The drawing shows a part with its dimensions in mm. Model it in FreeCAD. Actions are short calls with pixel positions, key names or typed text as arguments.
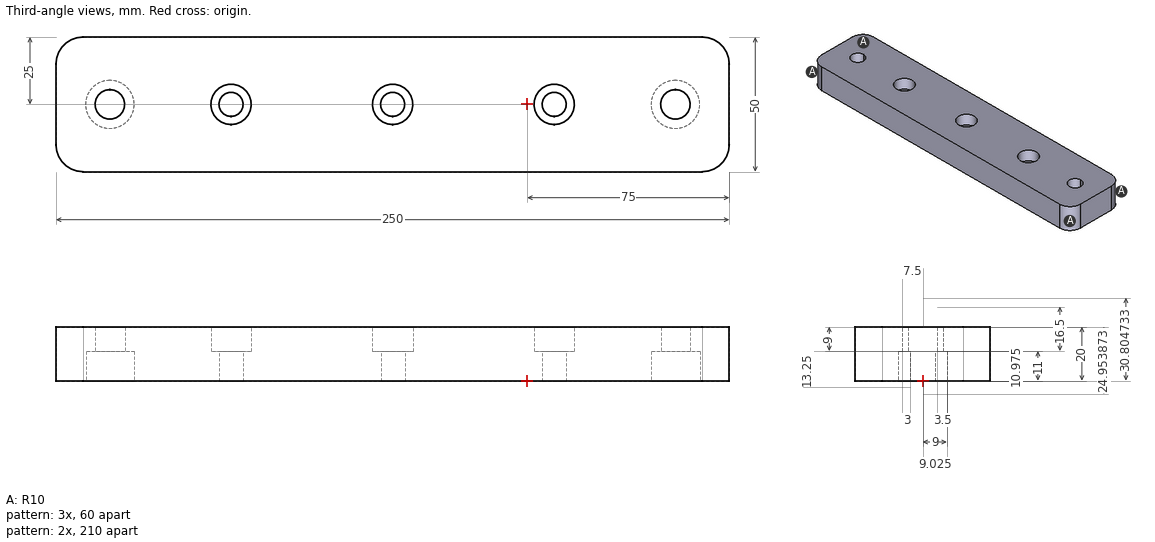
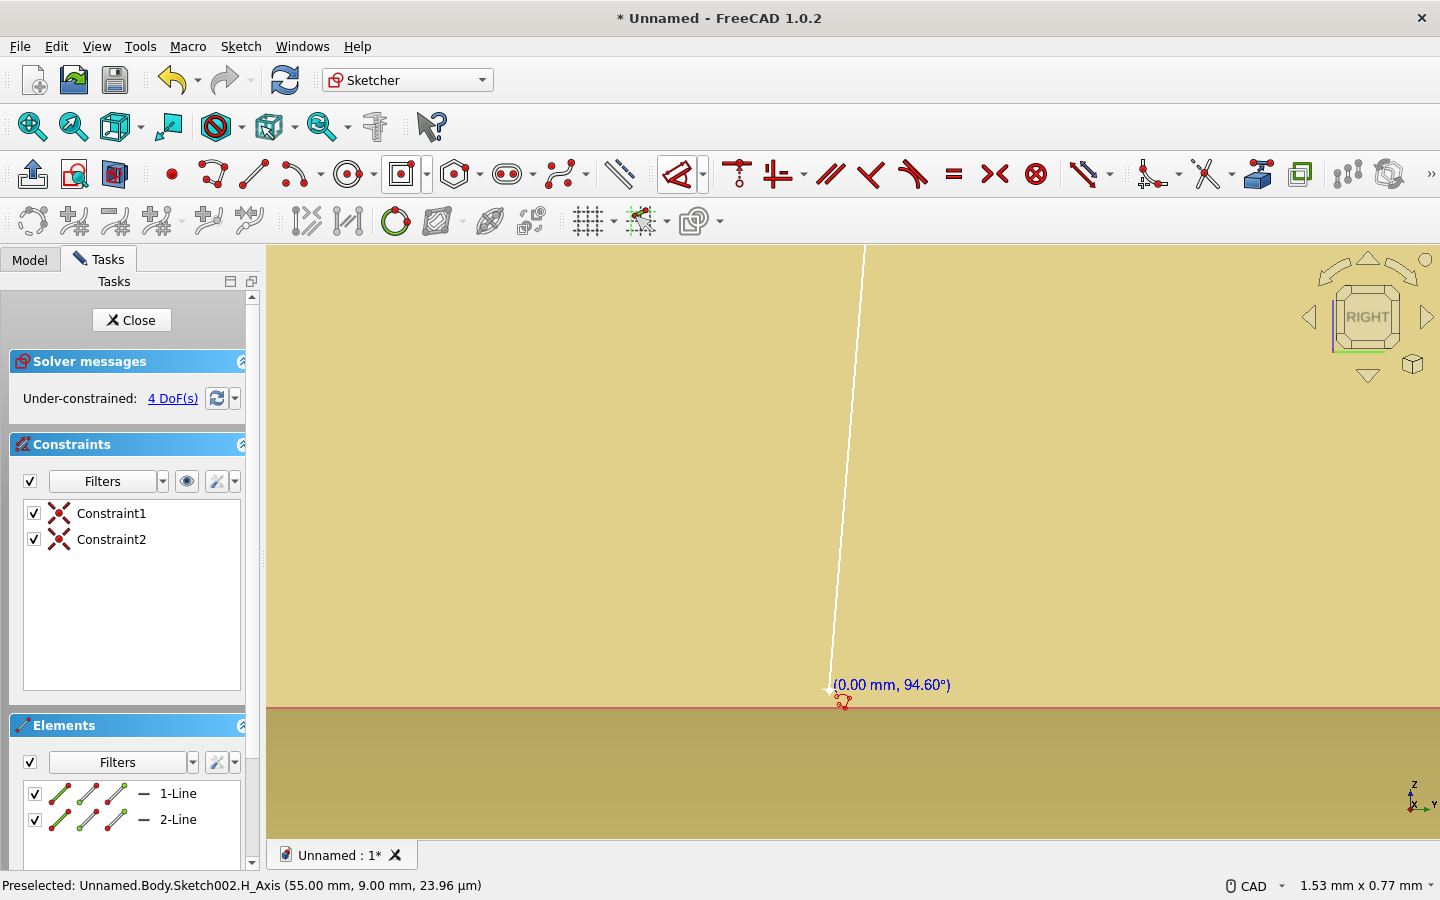
scroll(784, 542, down, 15)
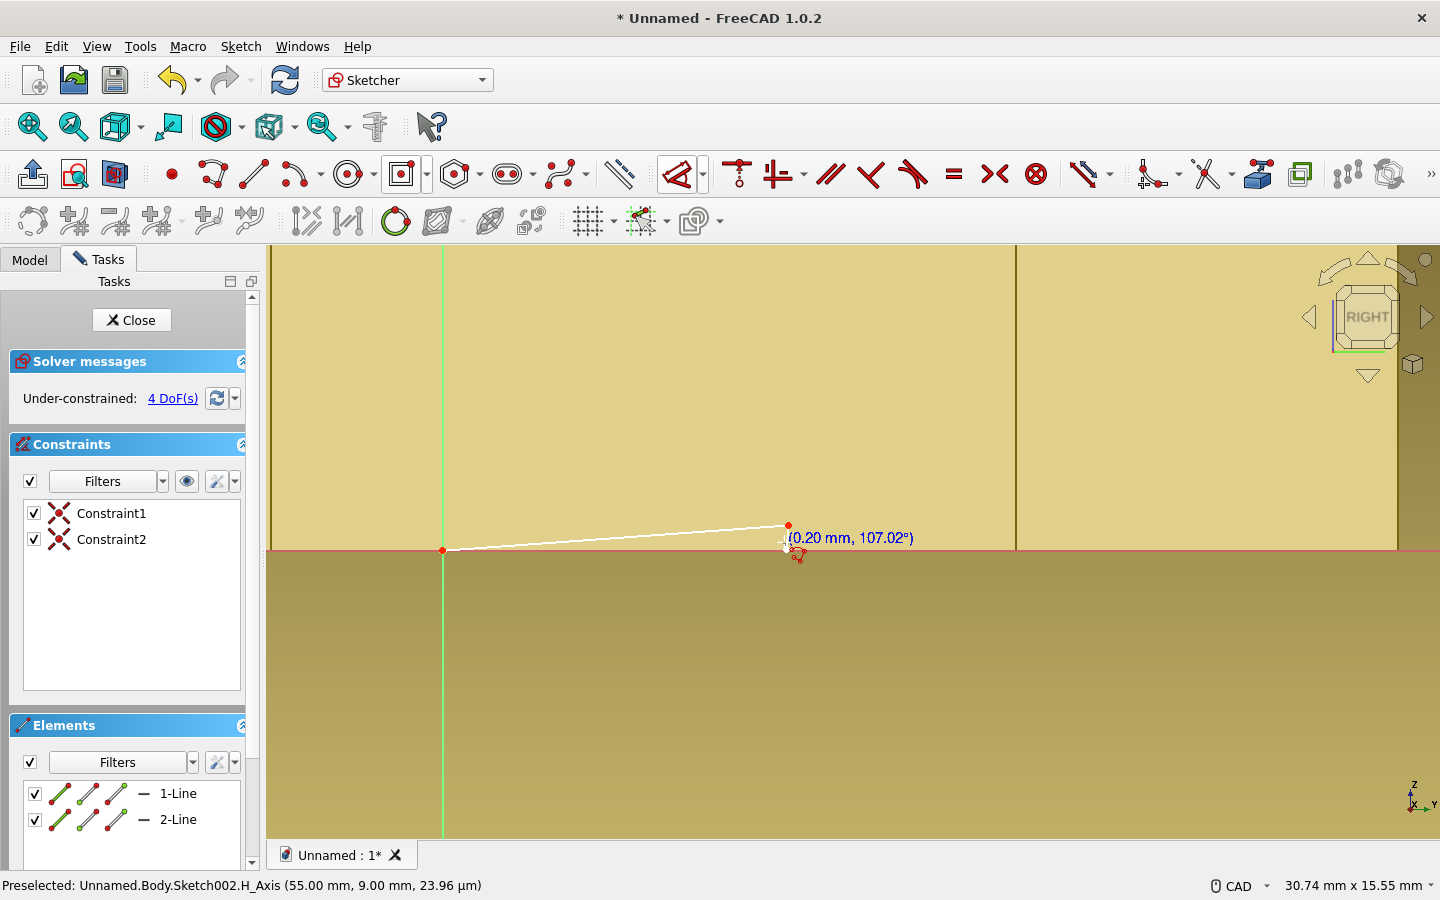
scroll(857, 792, down, 6)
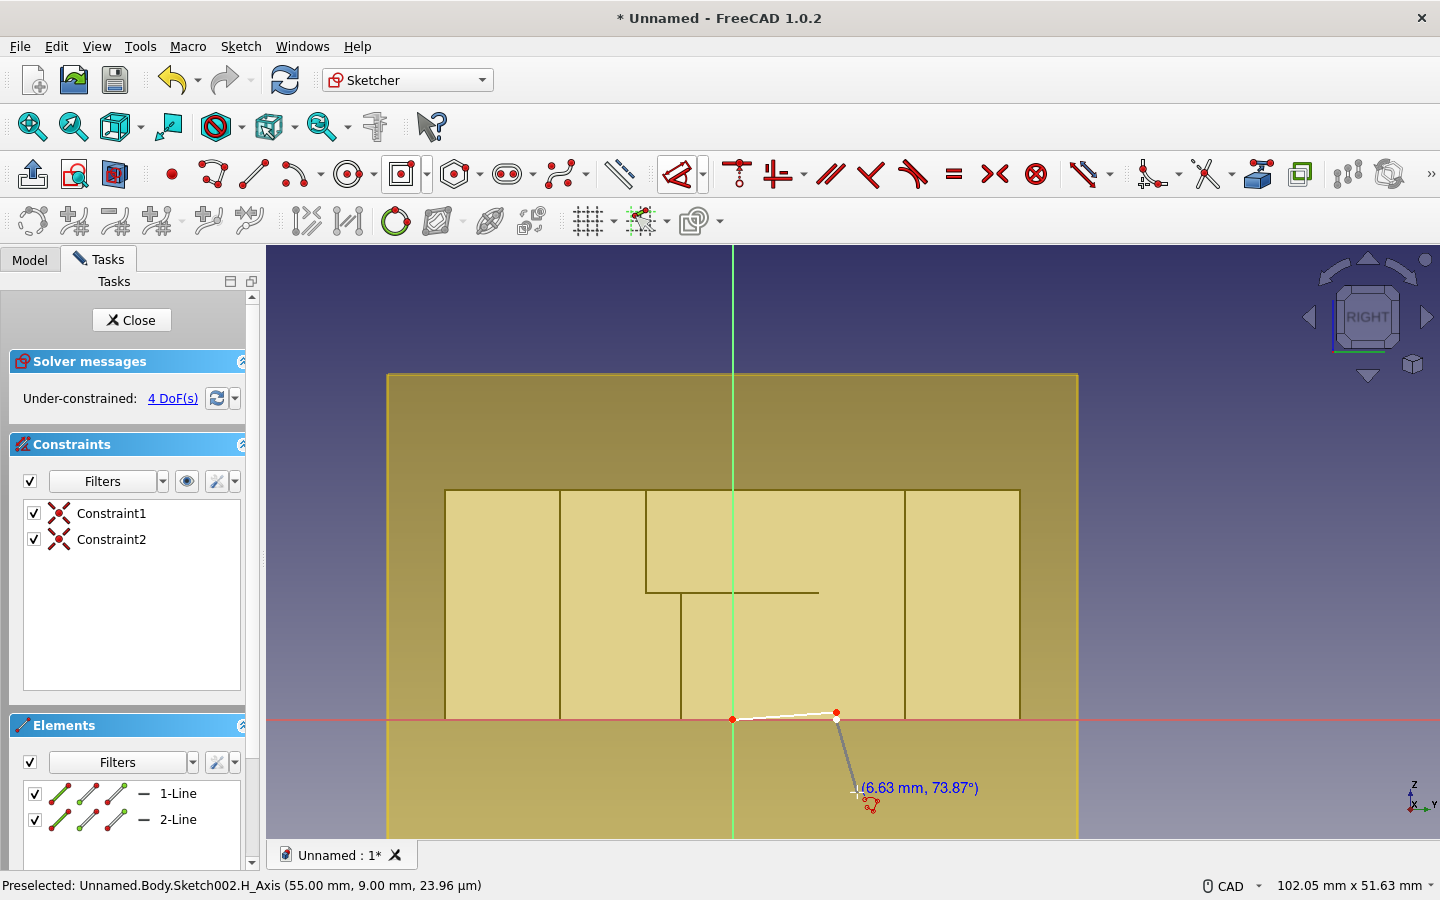
click(836, 593)
click(796, 593)
click(796, 404)
click(742, 366)
click(733, 720)
key(Escape)
key(Escape)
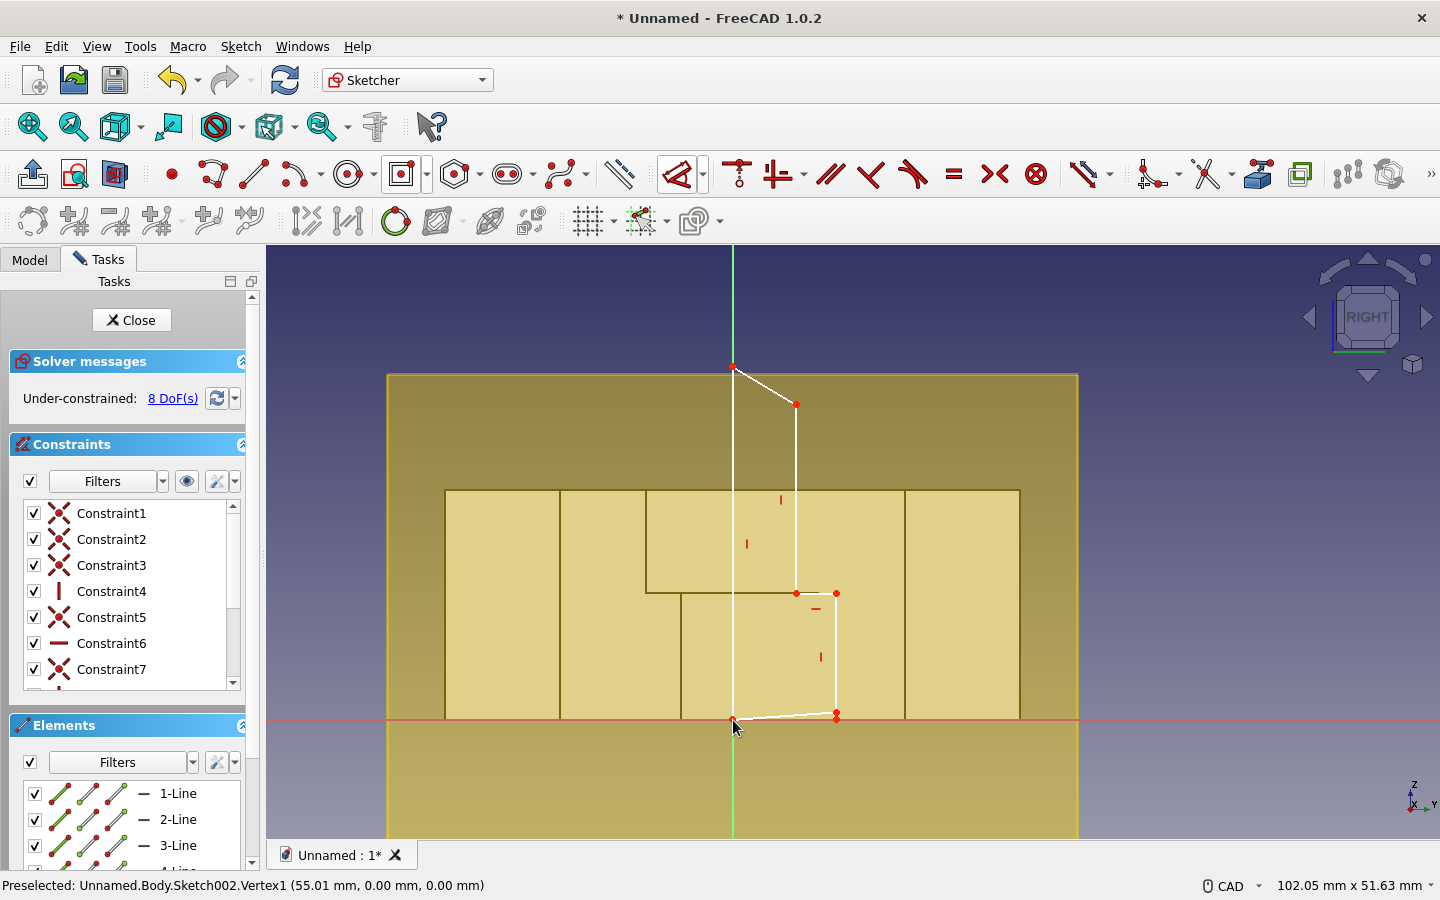
click(764, 718)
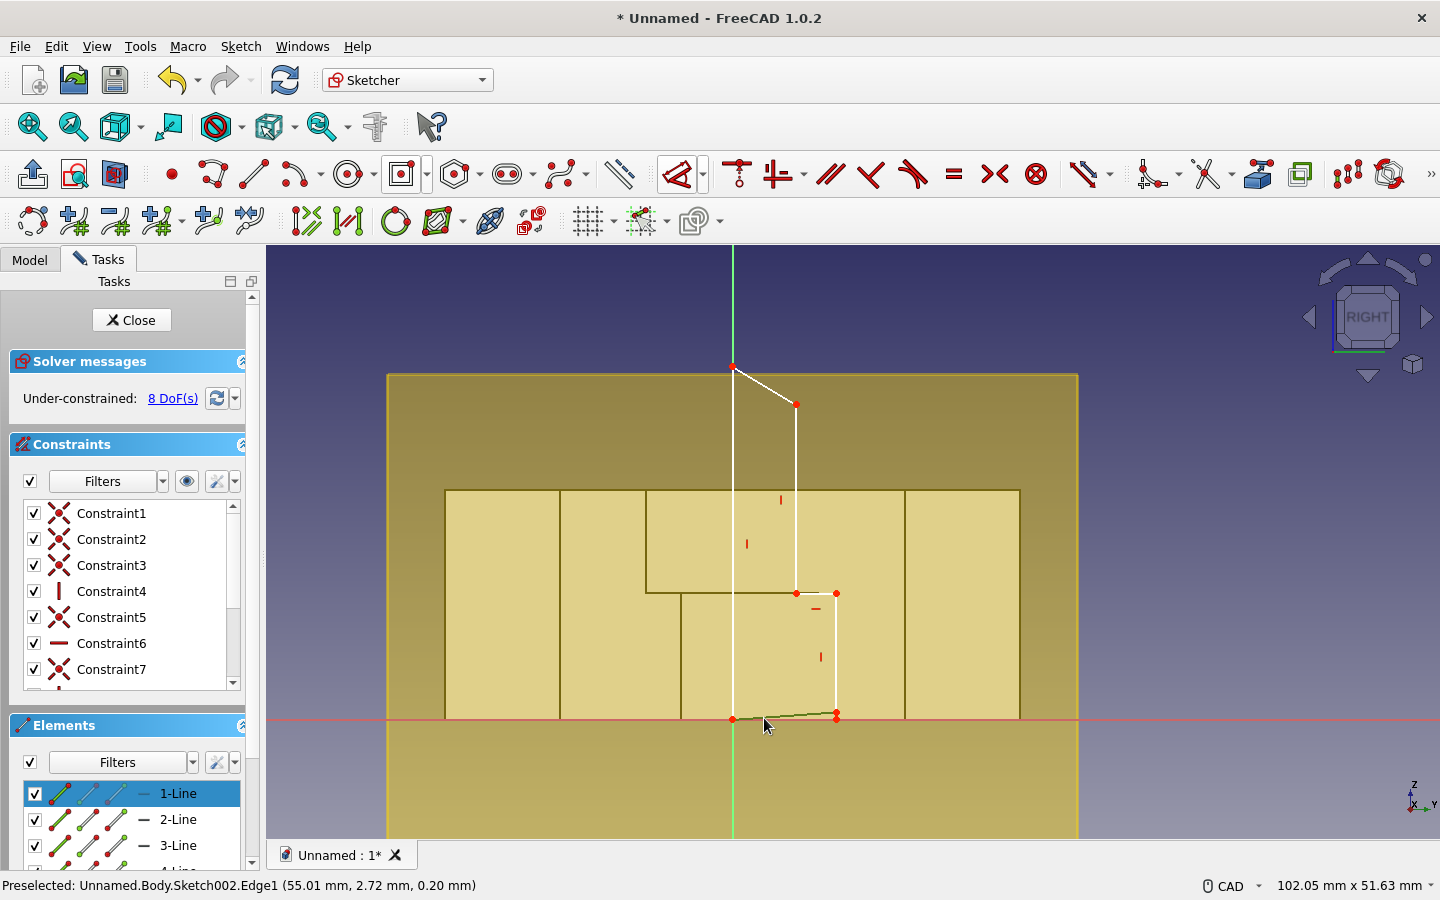
click(804, 174)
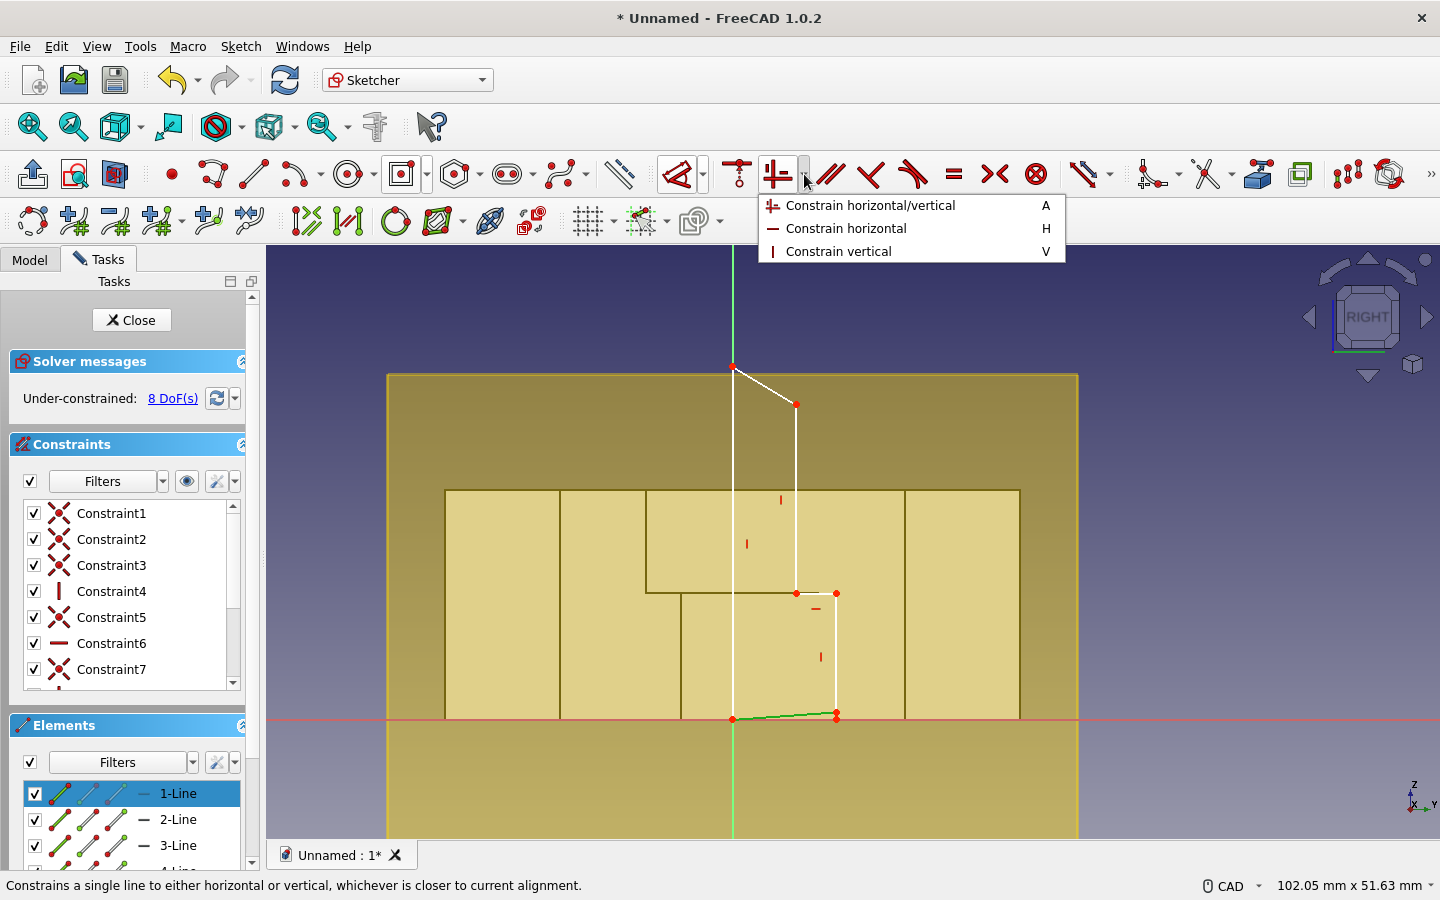
click(912, 228)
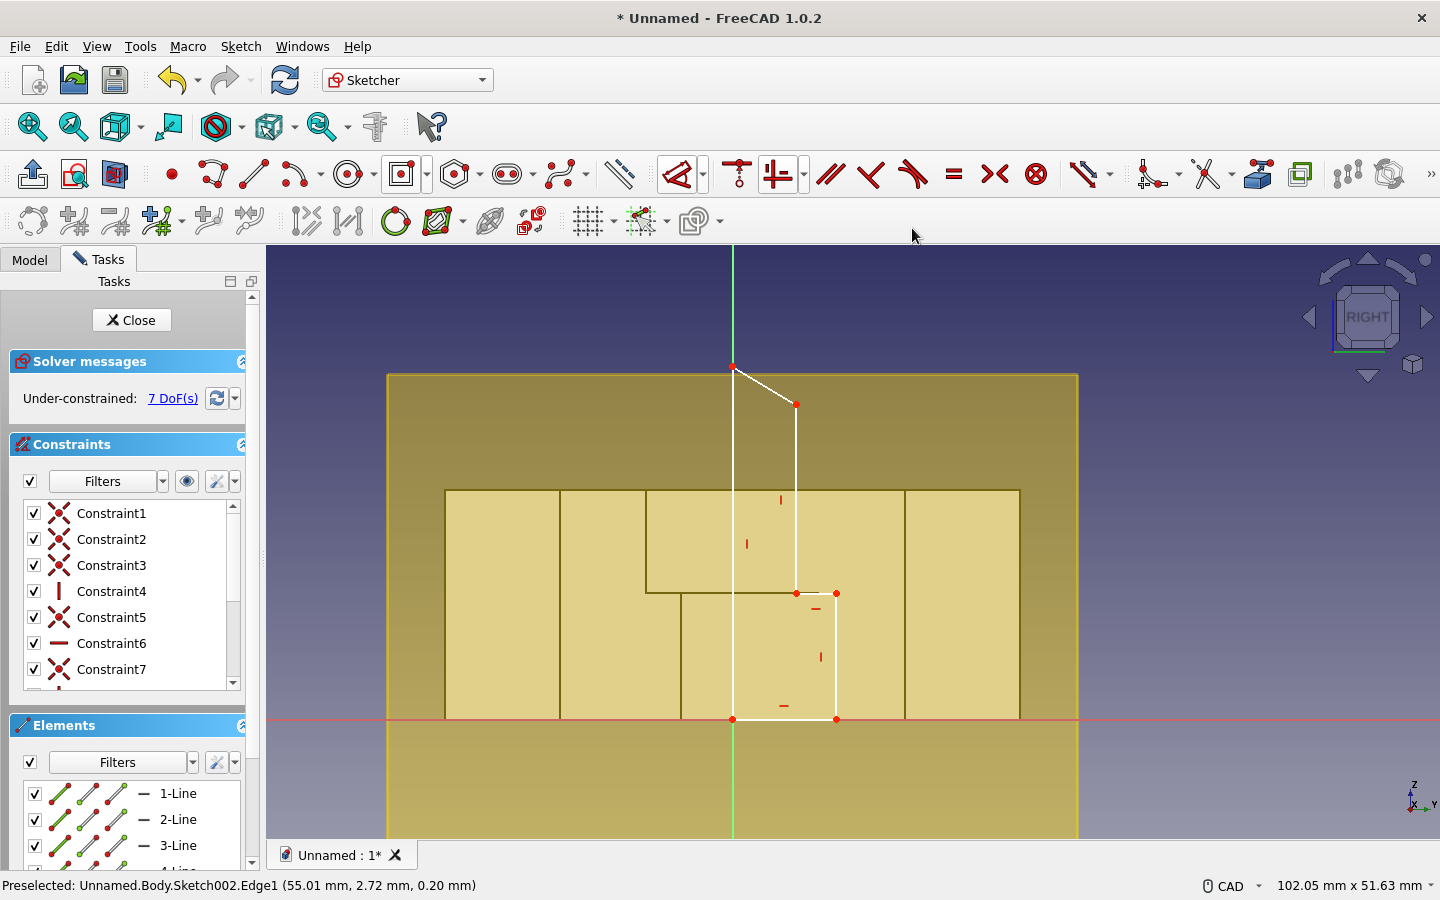
scroll(836, 720, up, 14)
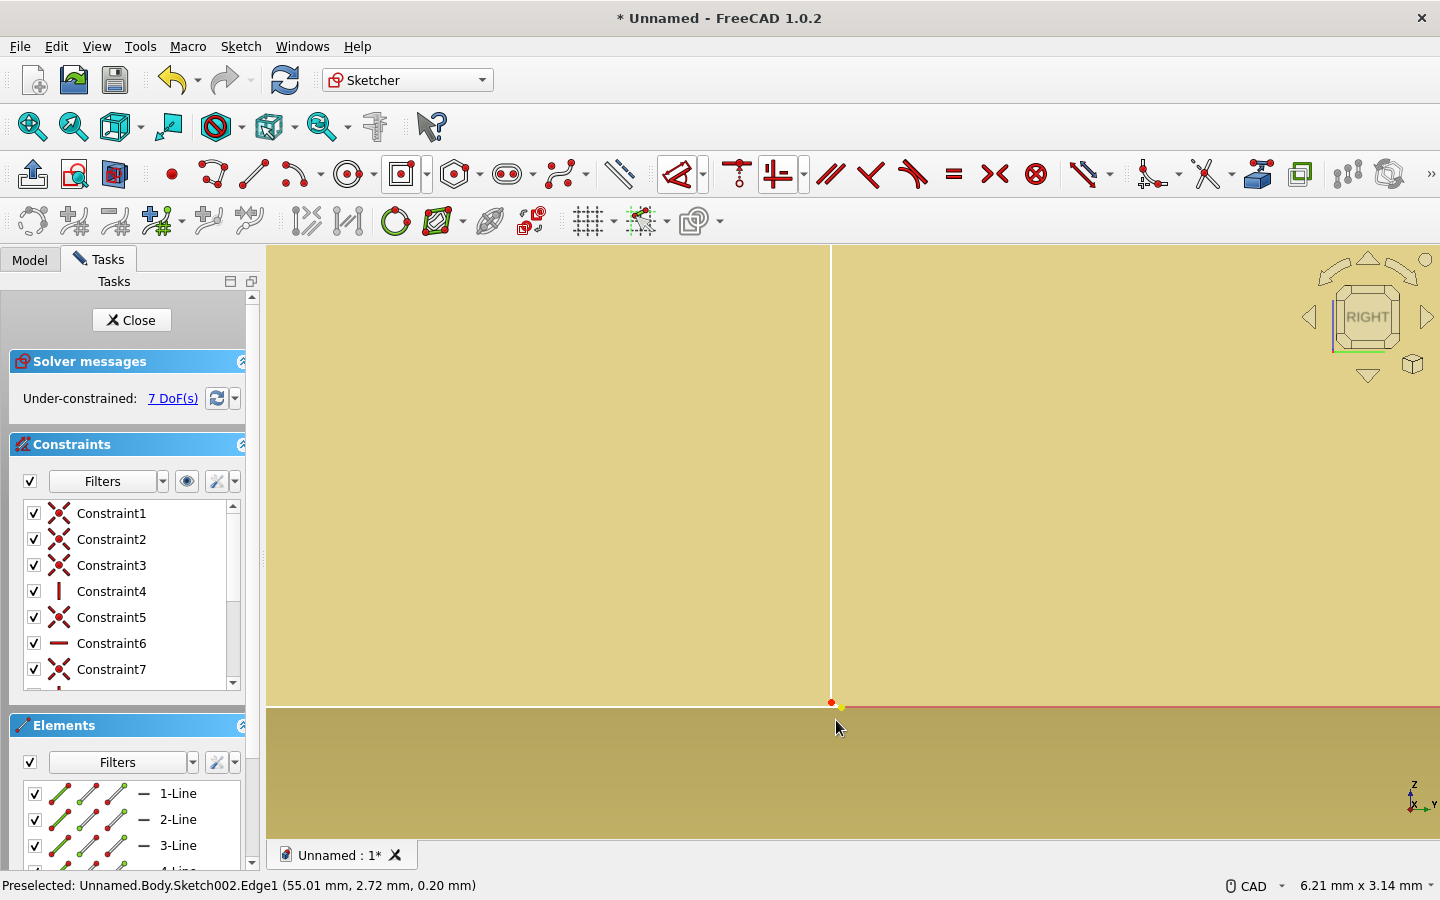
click(831, 703)